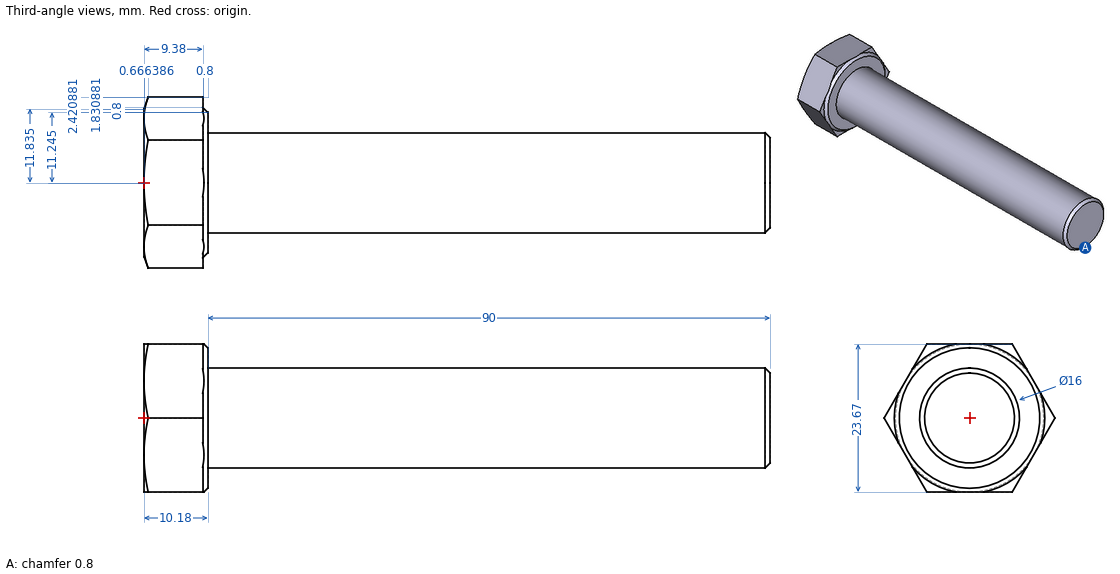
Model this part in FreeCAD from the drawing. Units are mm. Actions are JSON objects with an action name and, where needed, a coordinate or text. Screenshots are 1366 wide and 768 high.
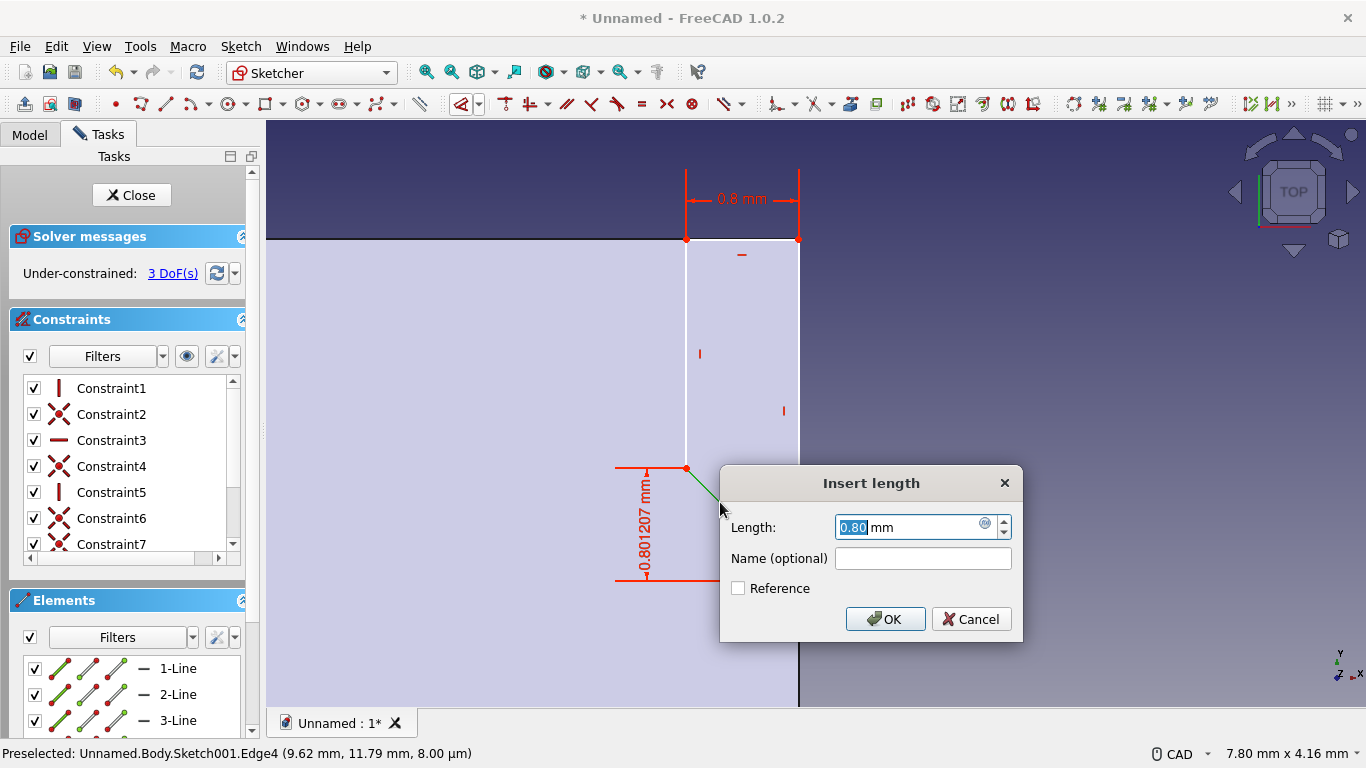
{"action": "type", "text": "0.8"}
{"action": "key", "text": "Return"}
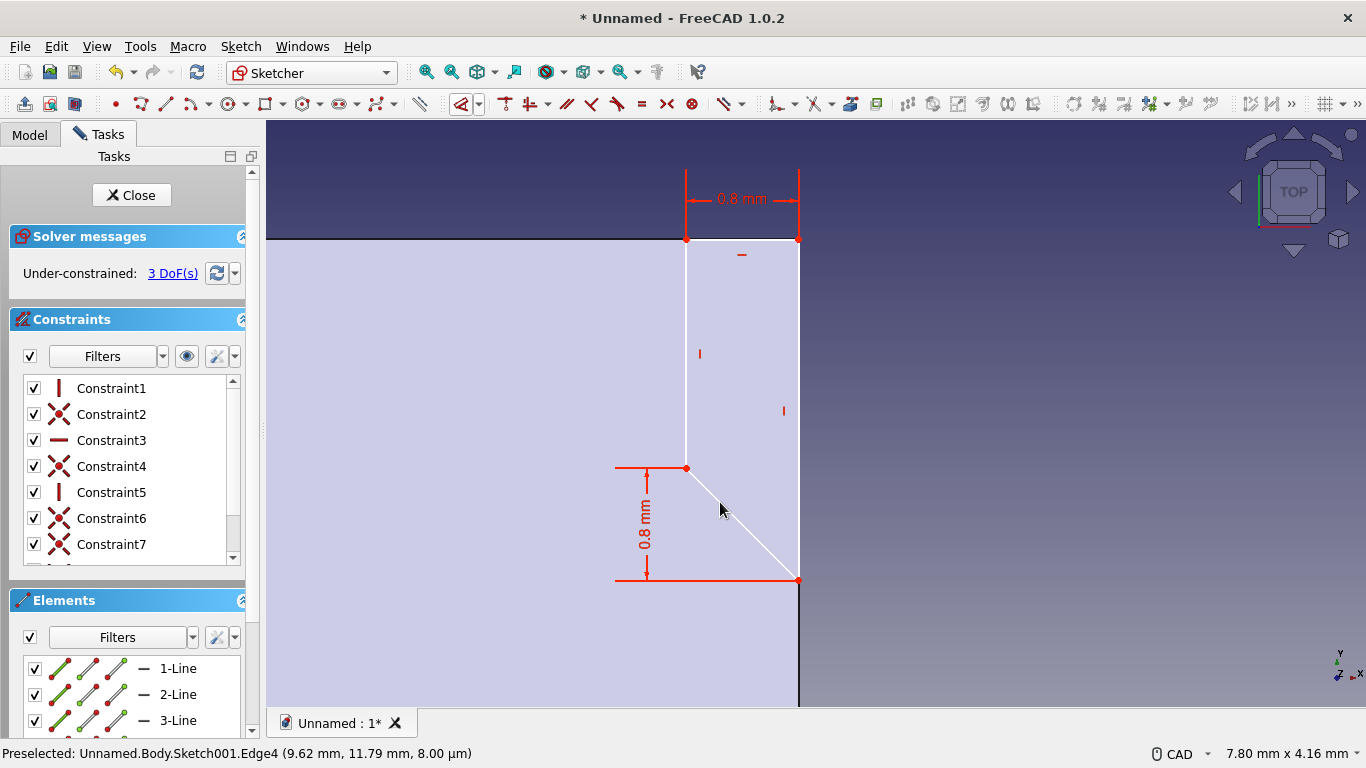
{"action": "left_click", "coordinate": [686, 240]}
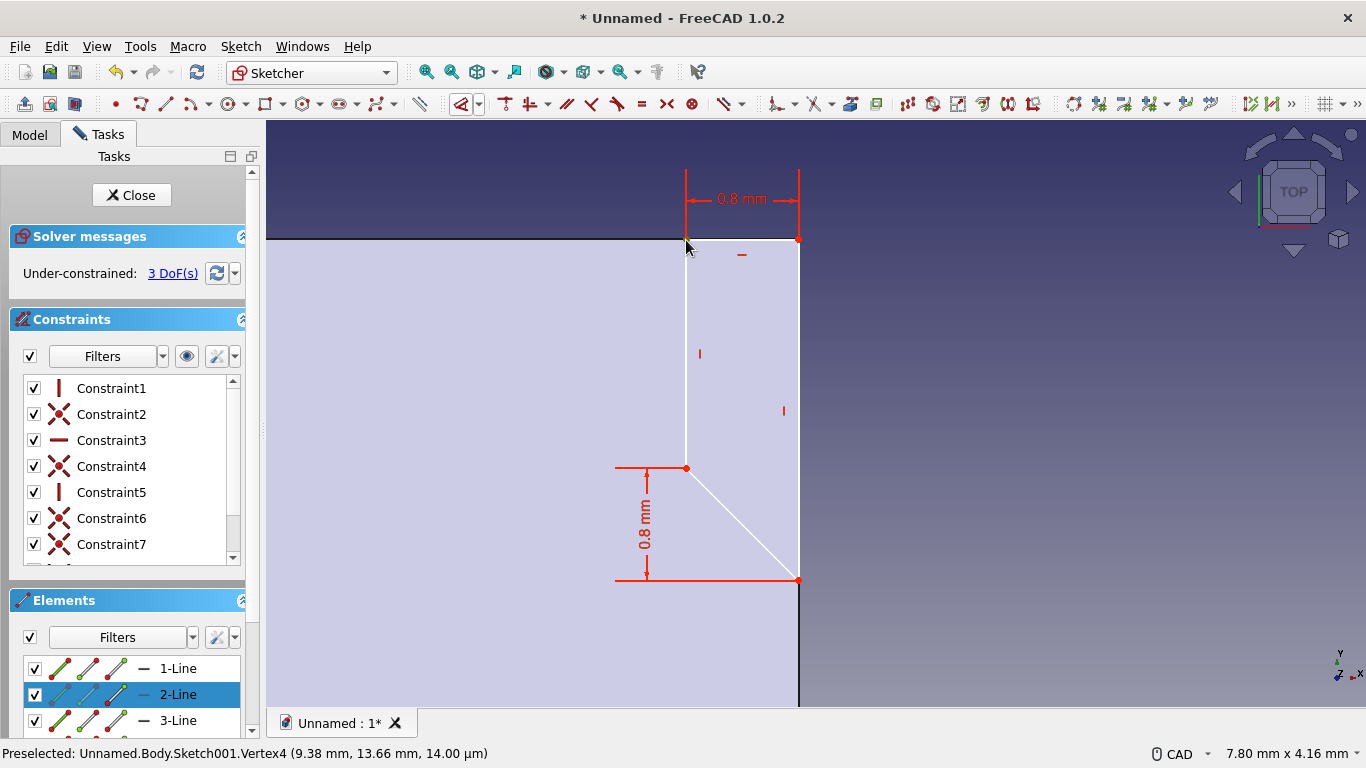
{"action": "key", "text": "l"}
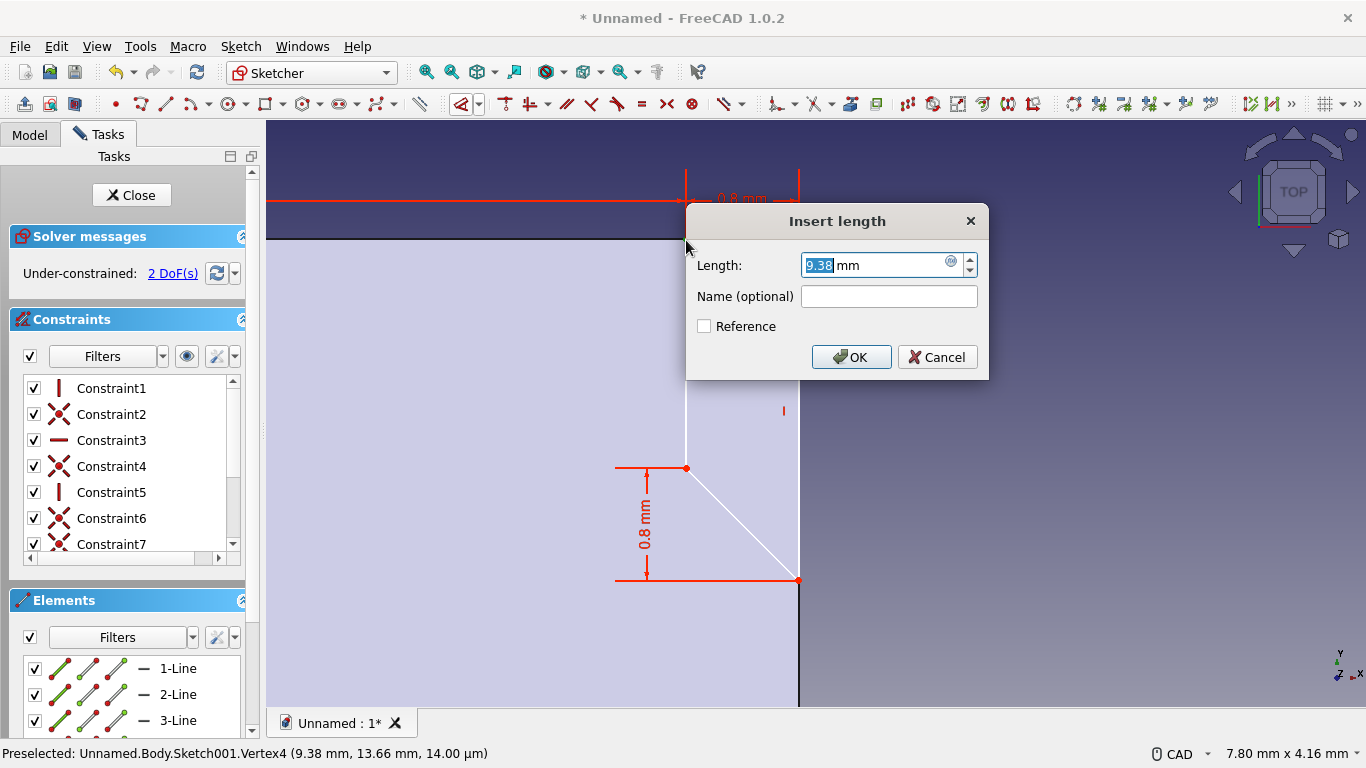
{"action": "type", "text": "9.38"}
{"action": "key", "text": "Return"}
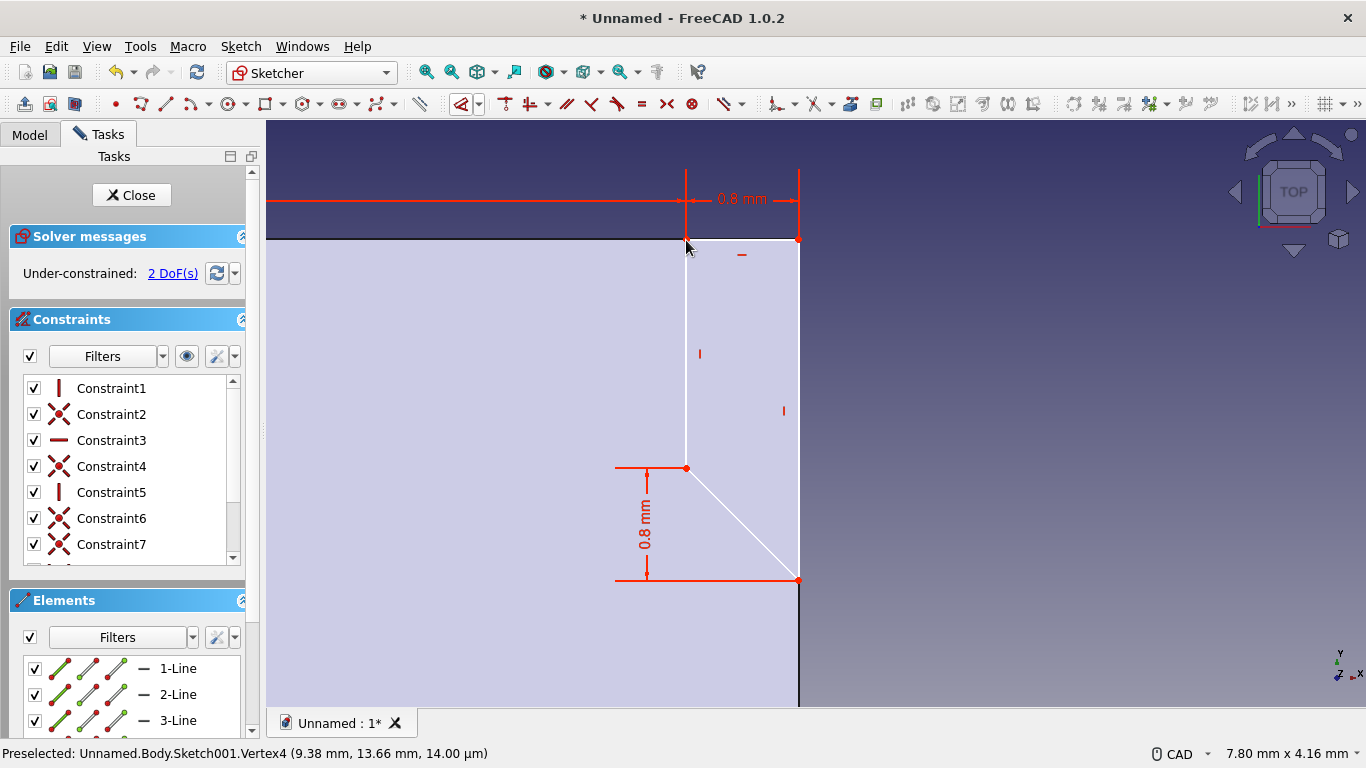
{"action": "left_click", "coordinate": [799, 581]}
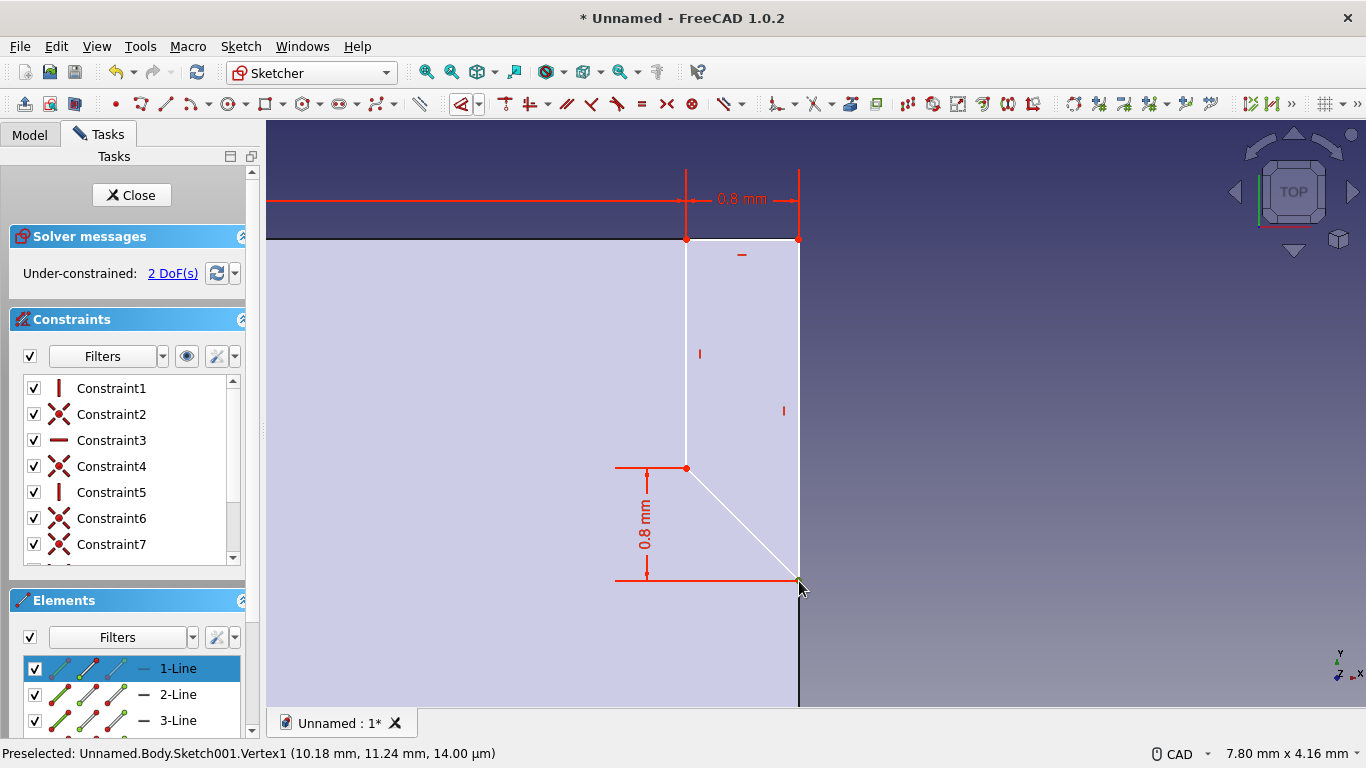
{"action": "key", "text": "i"}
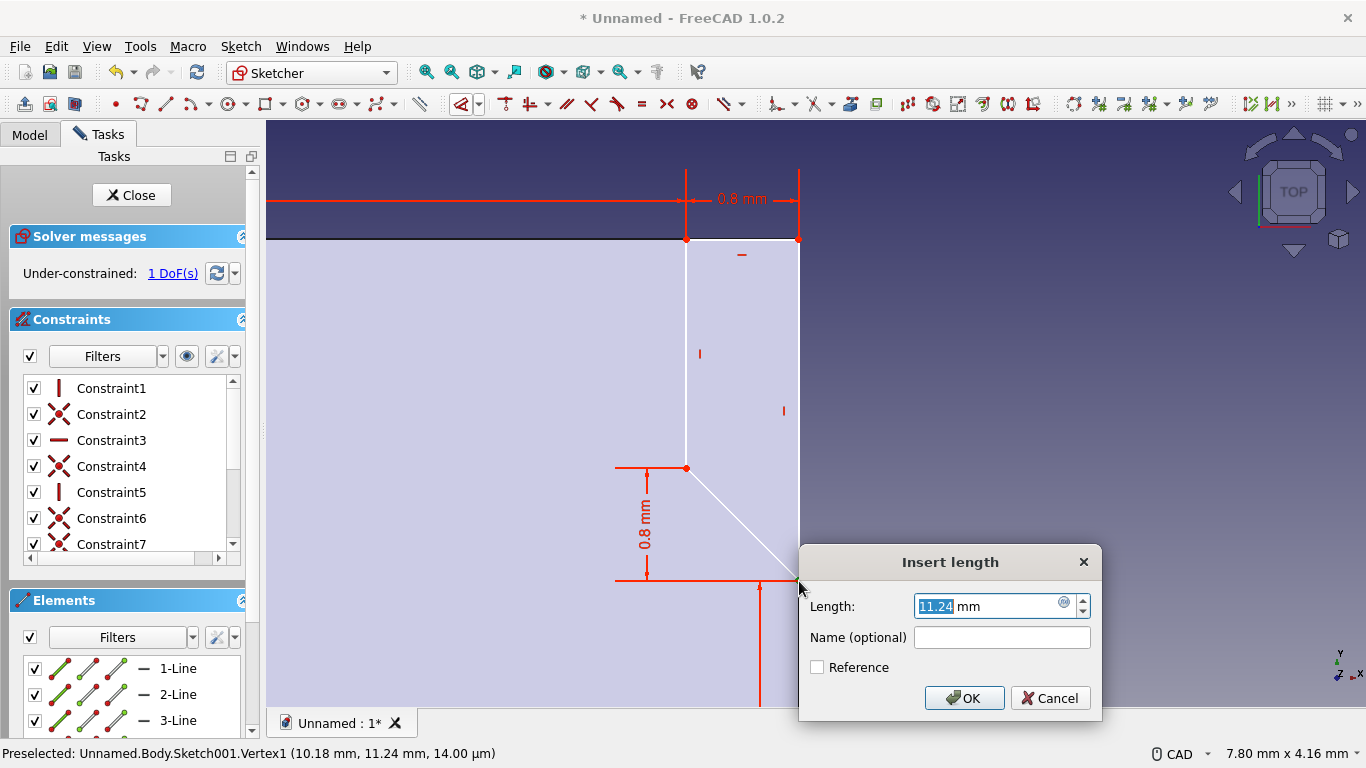
{"action": "type", "text": "11.245"}
{"action": "key", "text": "Return"}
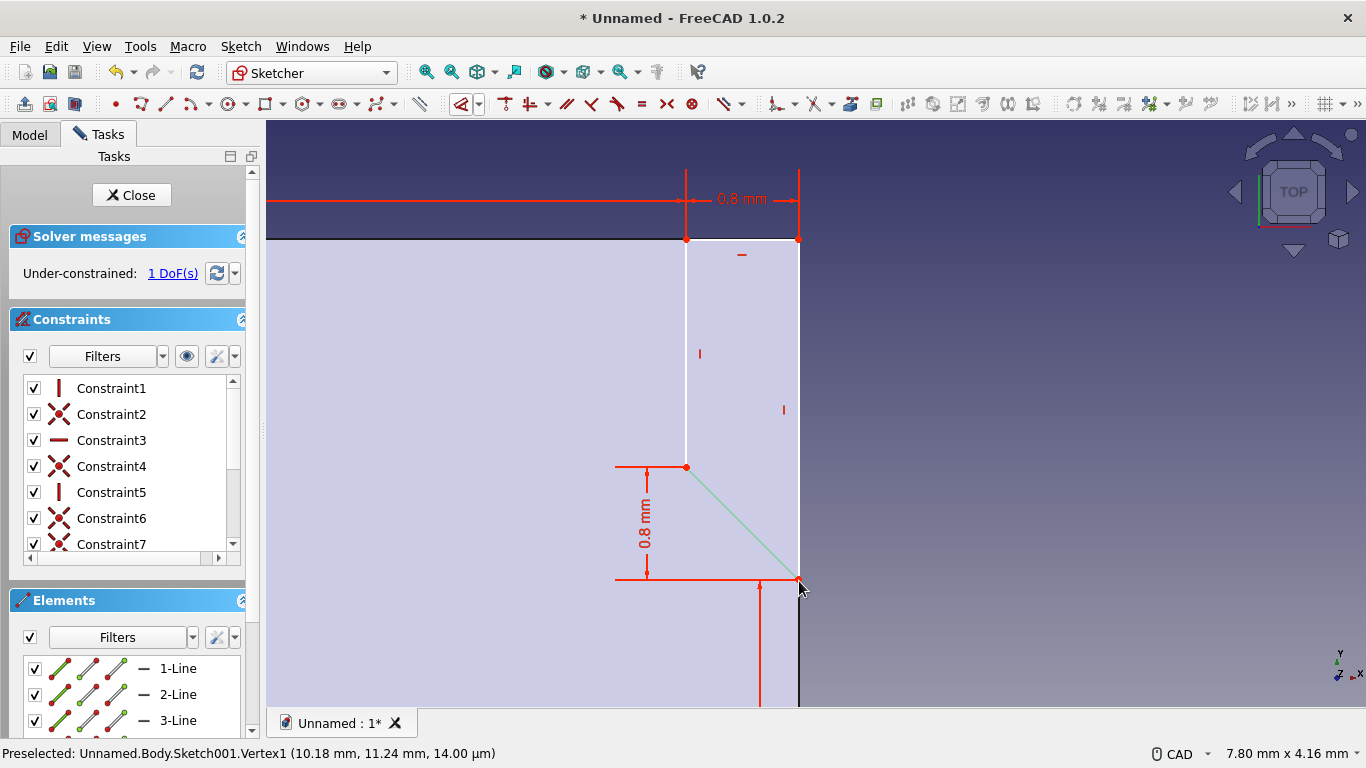
{"action": "left_click", "coordinate": [799, 478]}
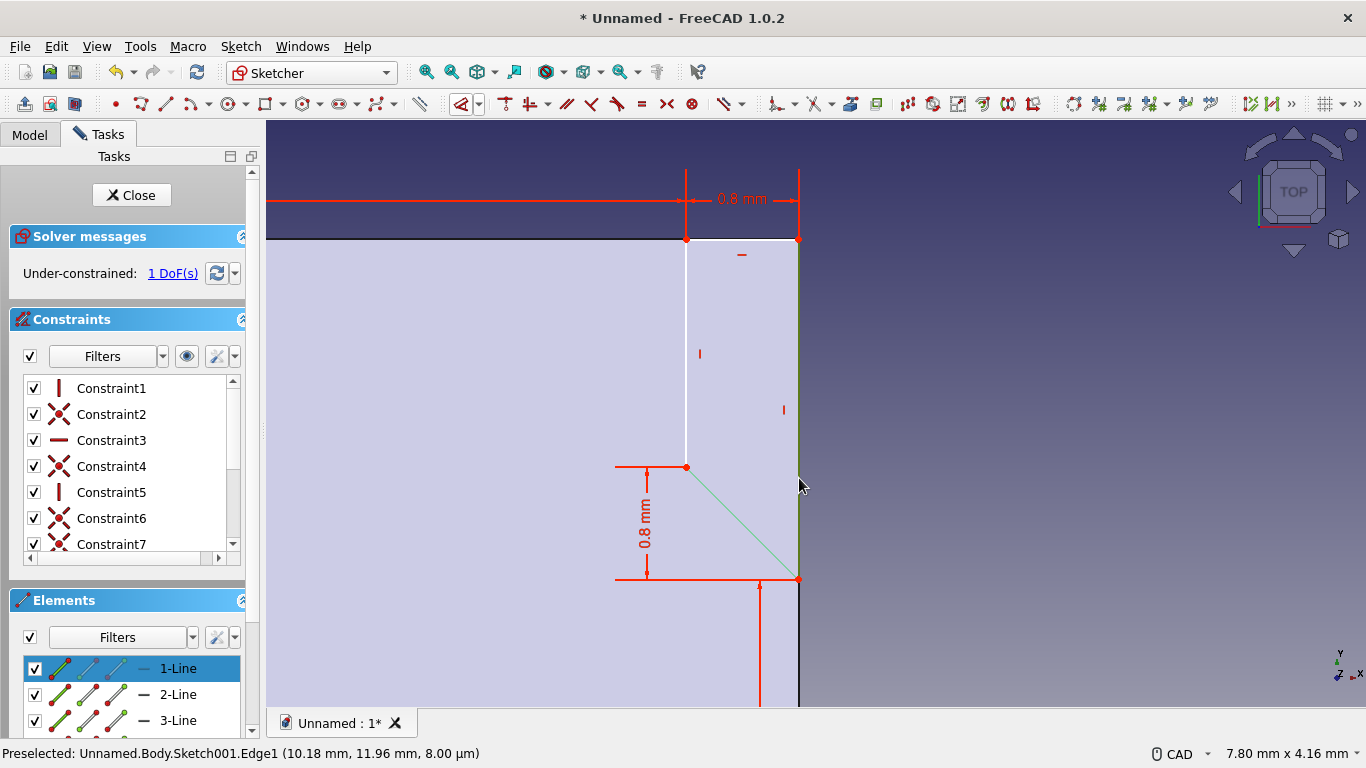
{"action": "key", "text": "i"}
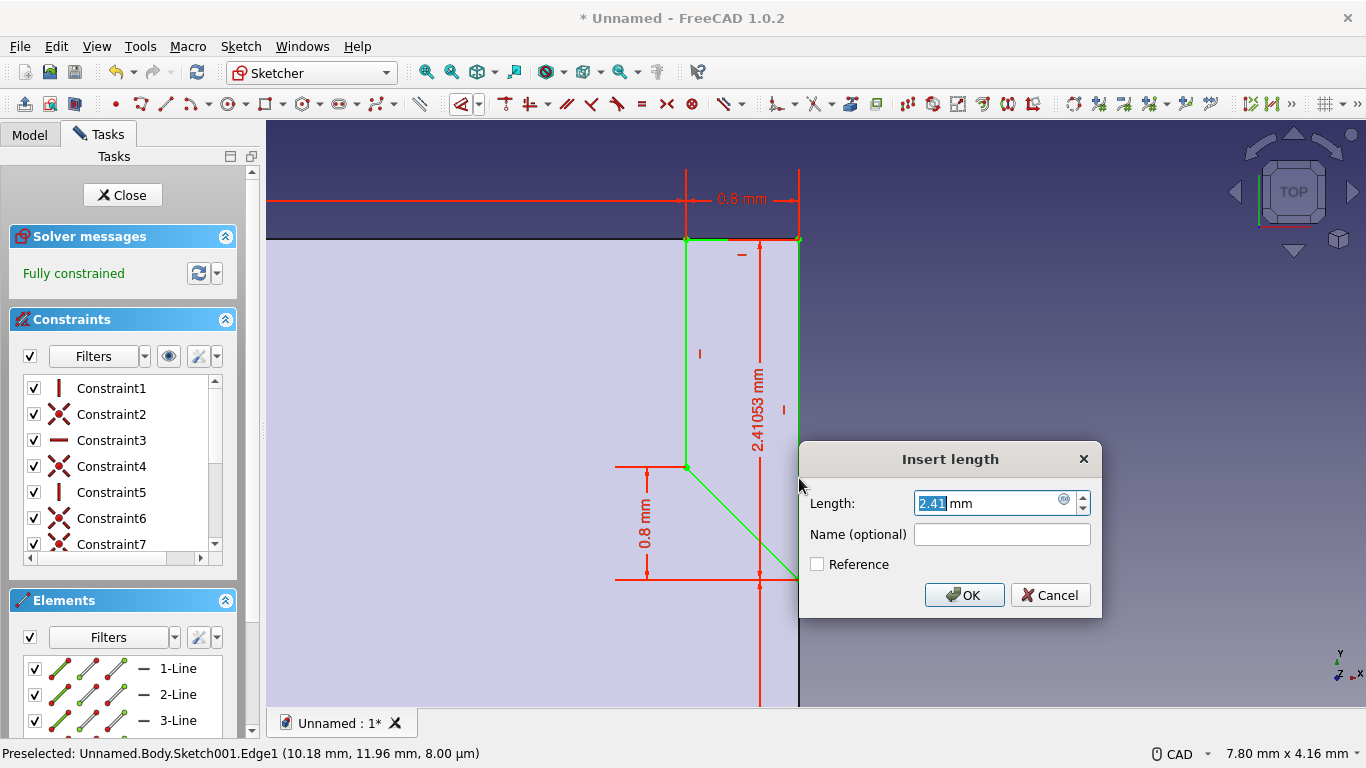
{"action": "type", "text": "2.420881"}
{"action": "key", "text": "Return"}